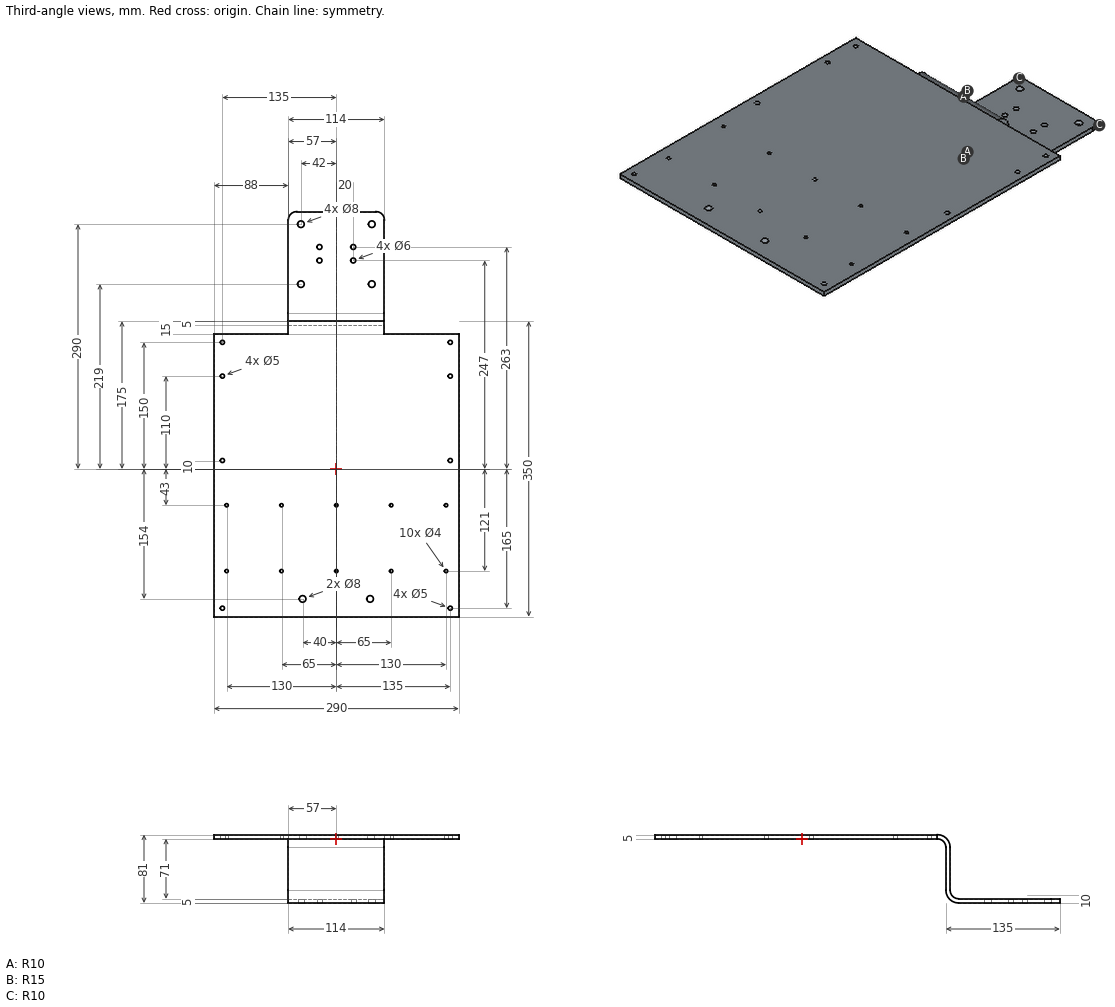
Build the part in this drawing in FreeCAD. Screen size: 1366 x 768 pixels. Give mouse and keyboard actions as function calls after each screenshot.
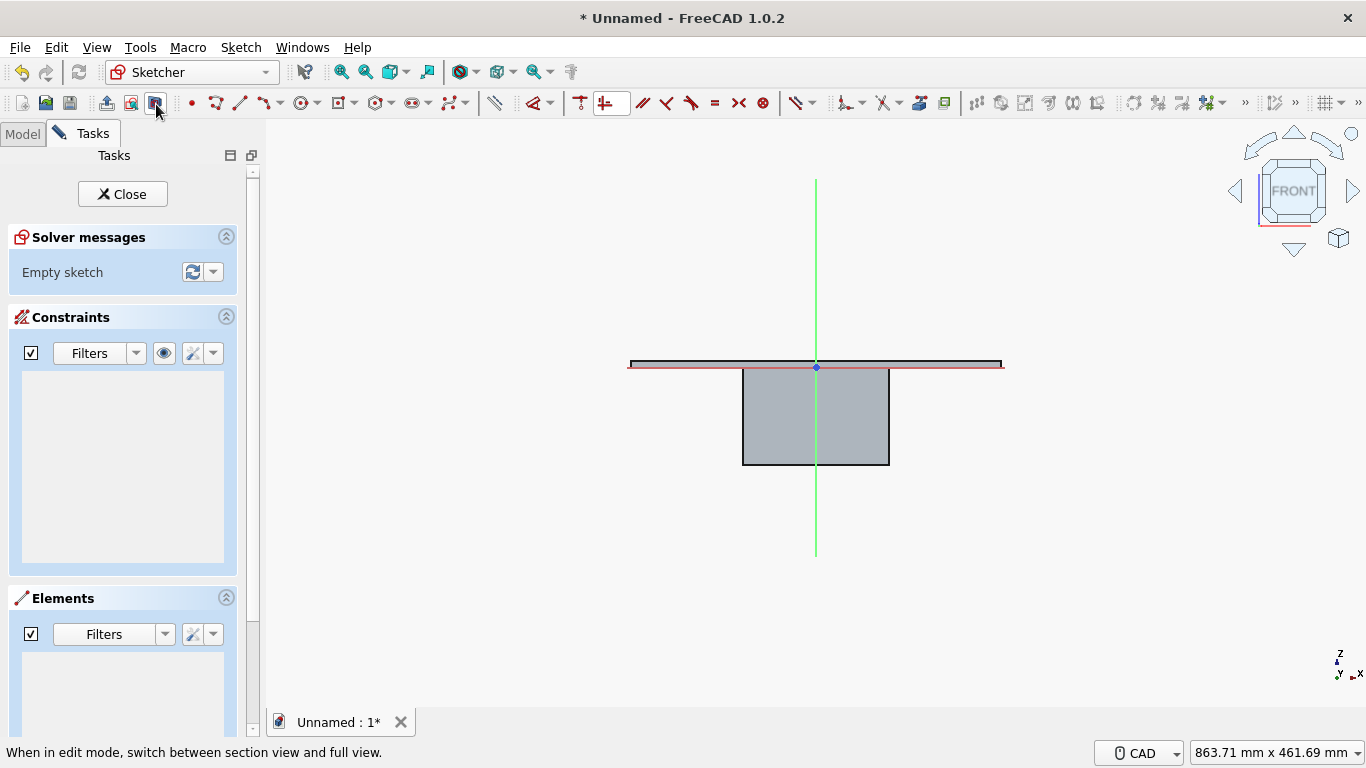
scroll(838, 417, up, 7)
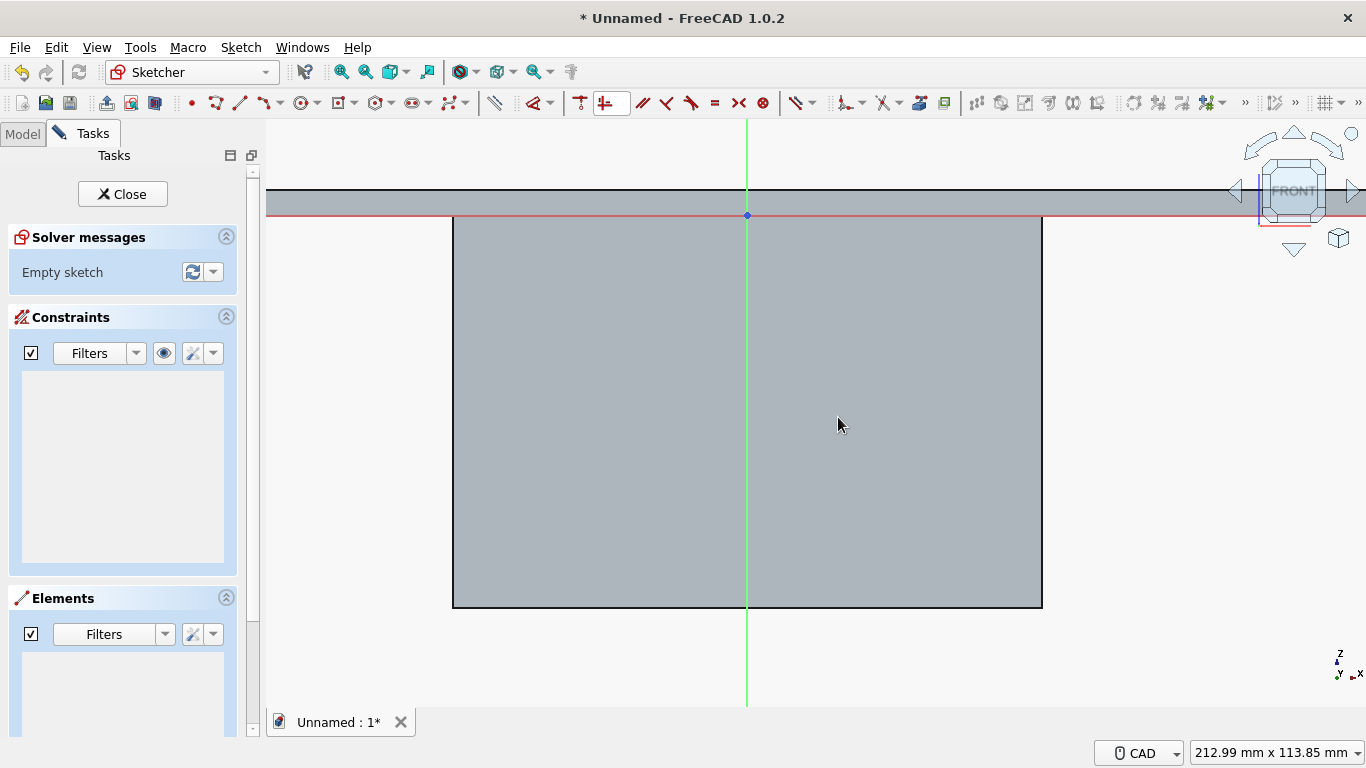
key(g)
key(r)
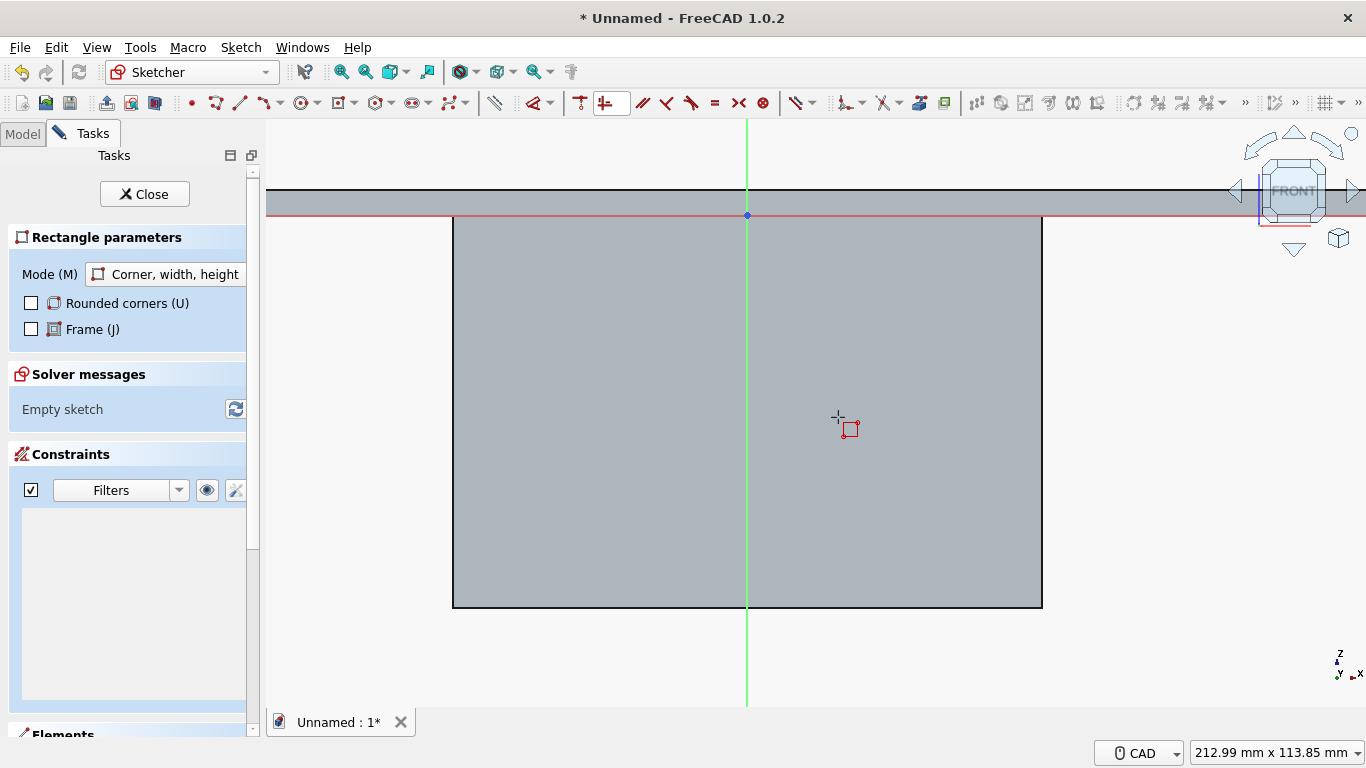
click(453, 583)
click(1042, 608)
key(Escape)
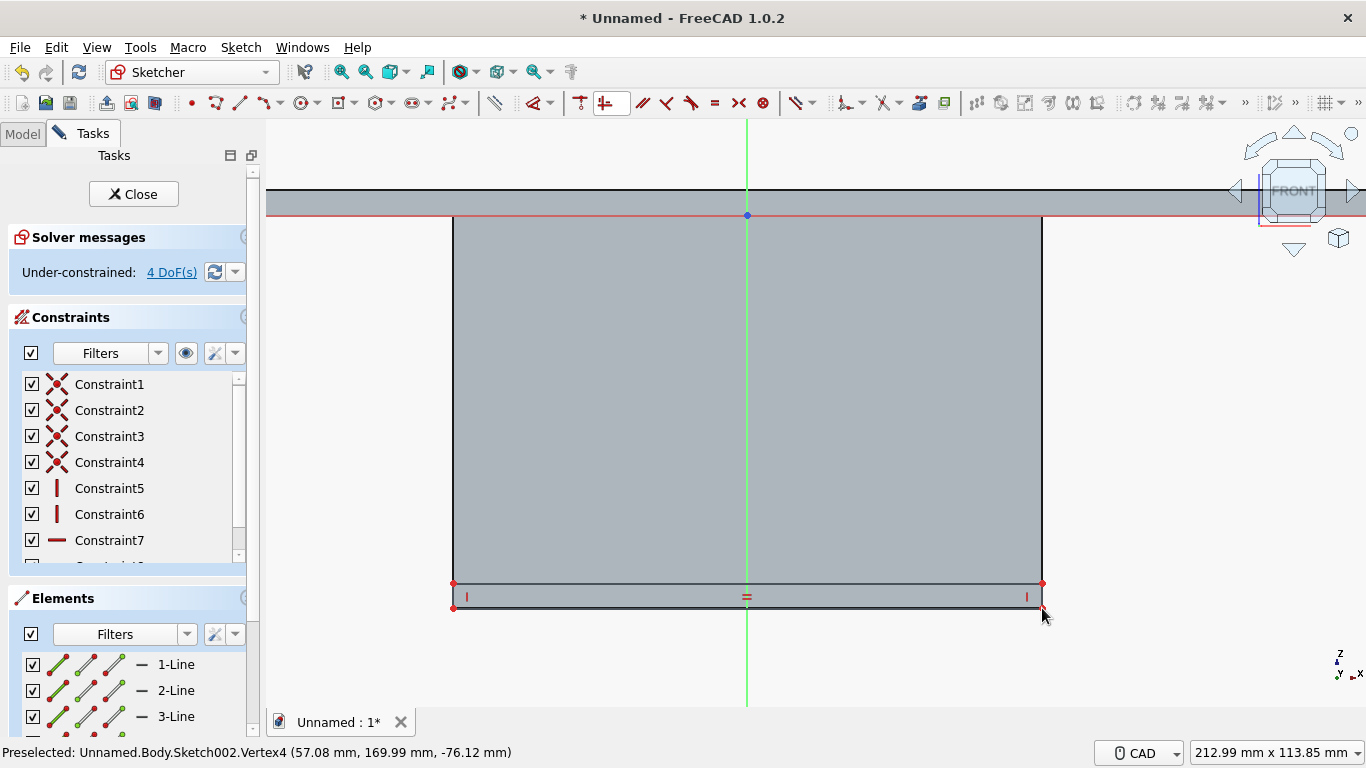
click(534, 104)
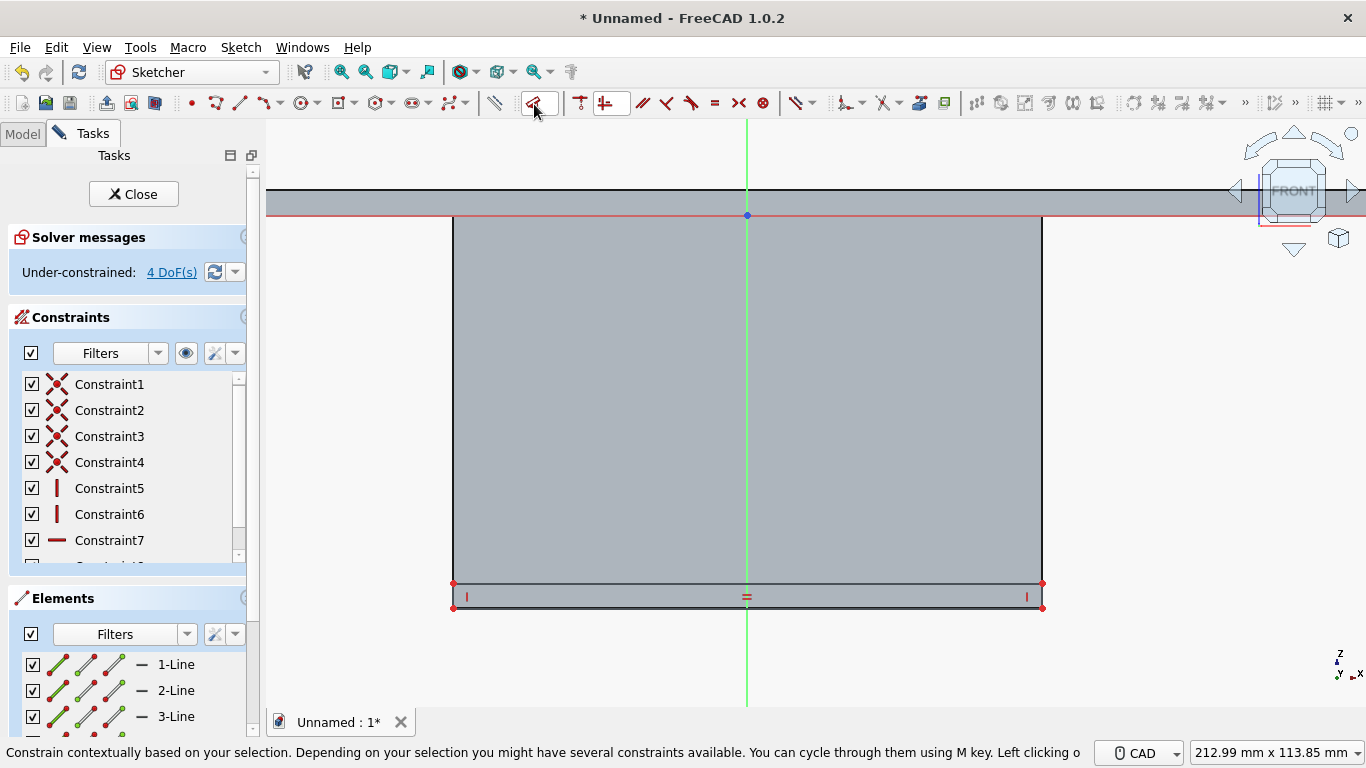
scroll(453, 594, up, 3)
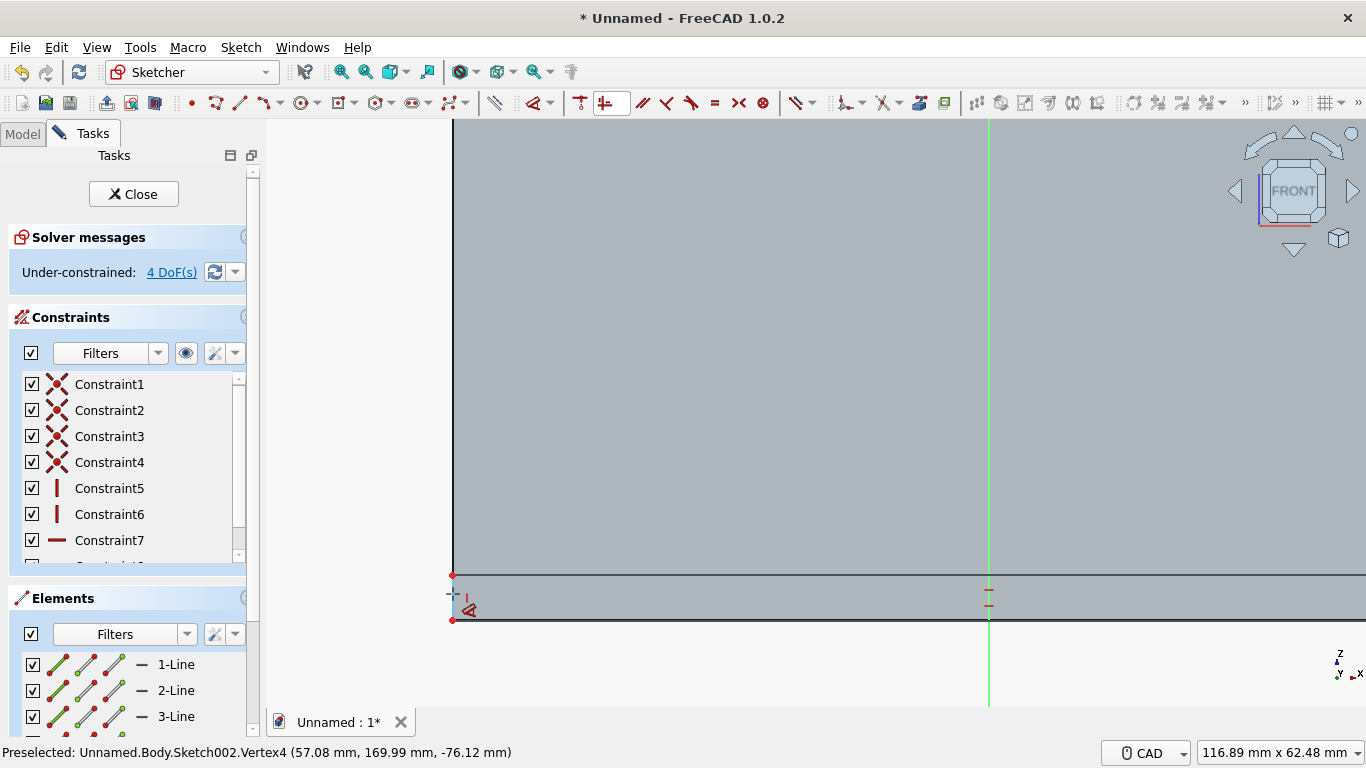
click(453, 593)
click(419, 598)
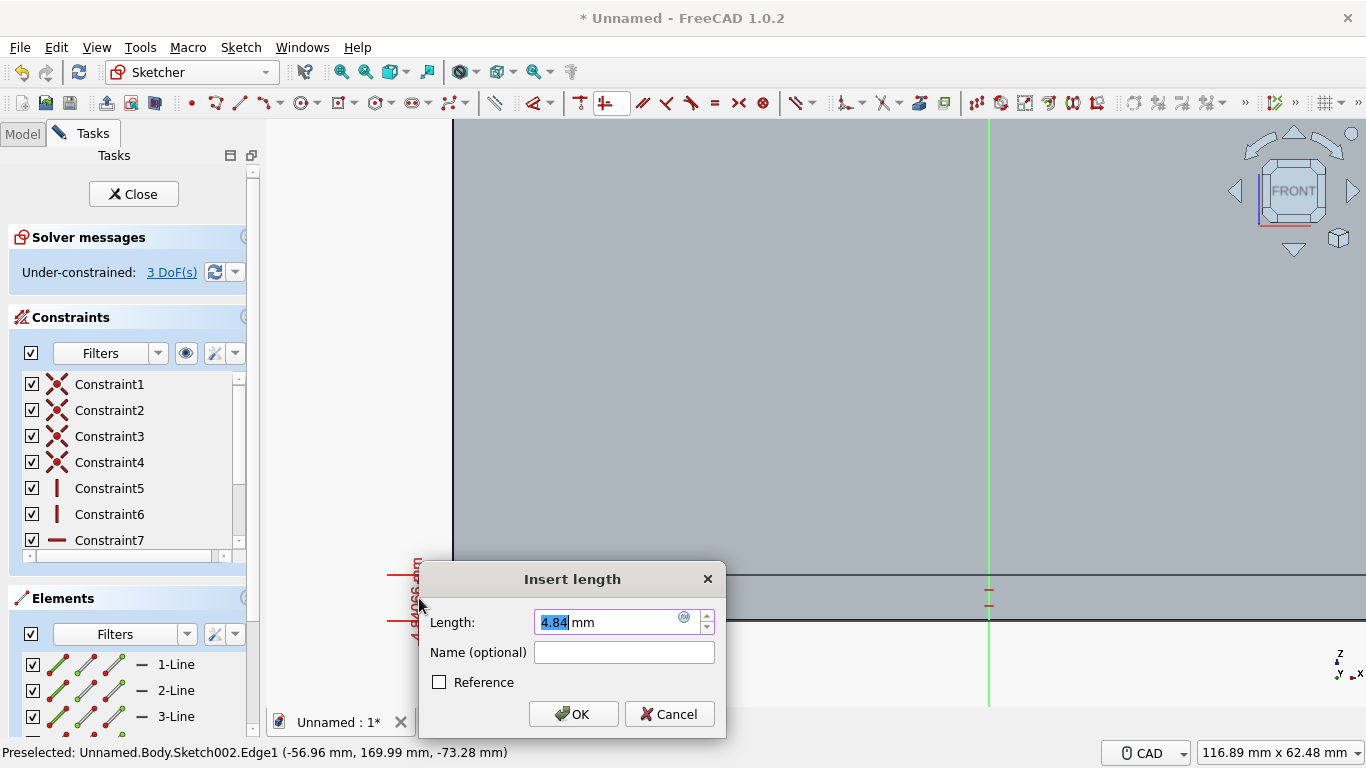
text(5)
key(Return)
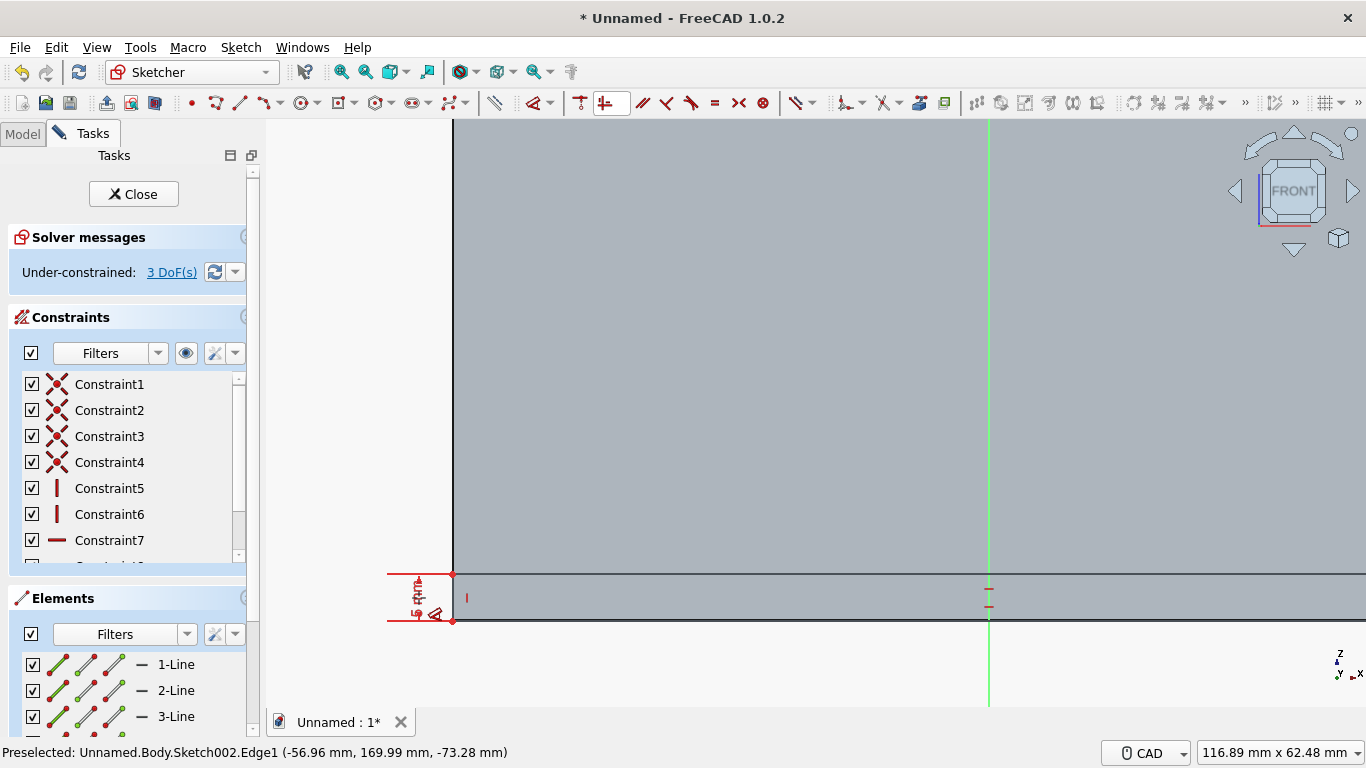
click(775, 621)
click(827, 655)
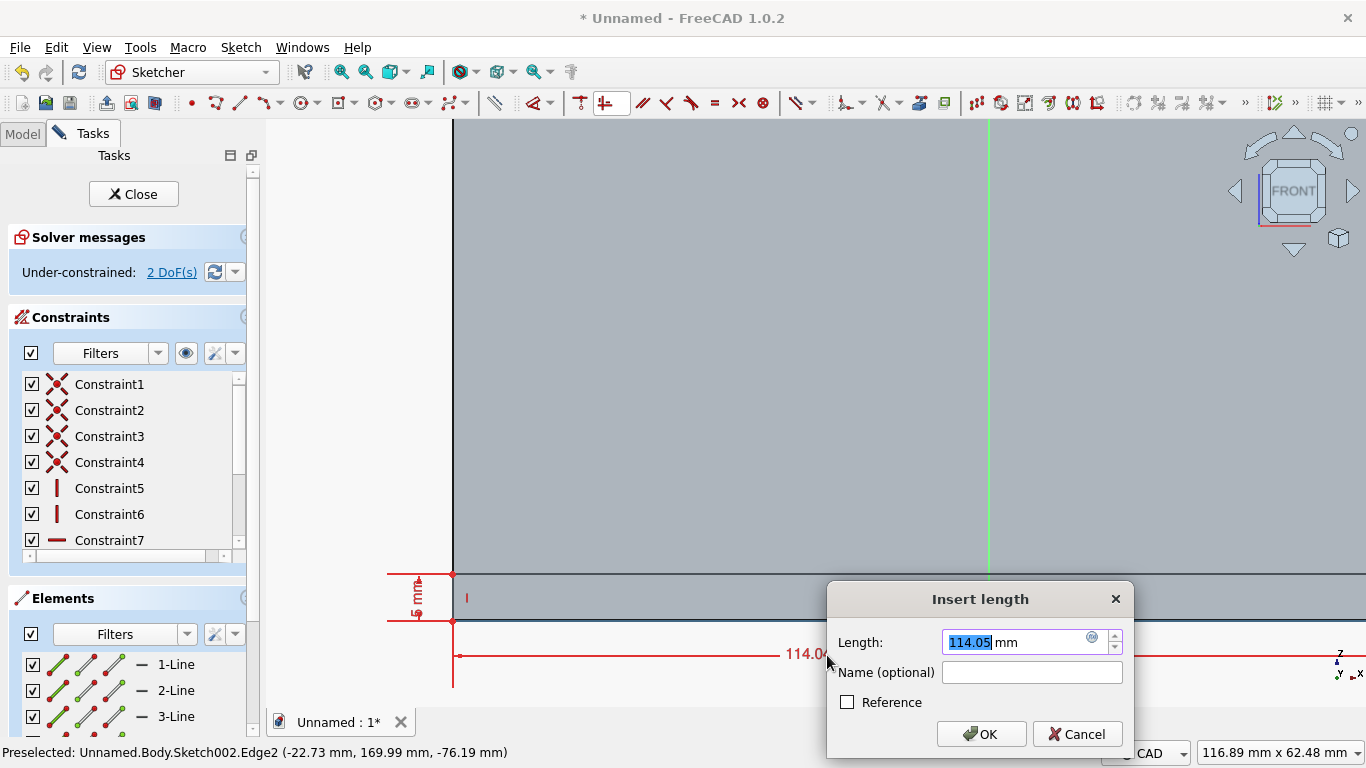
text(114)
key(Return)